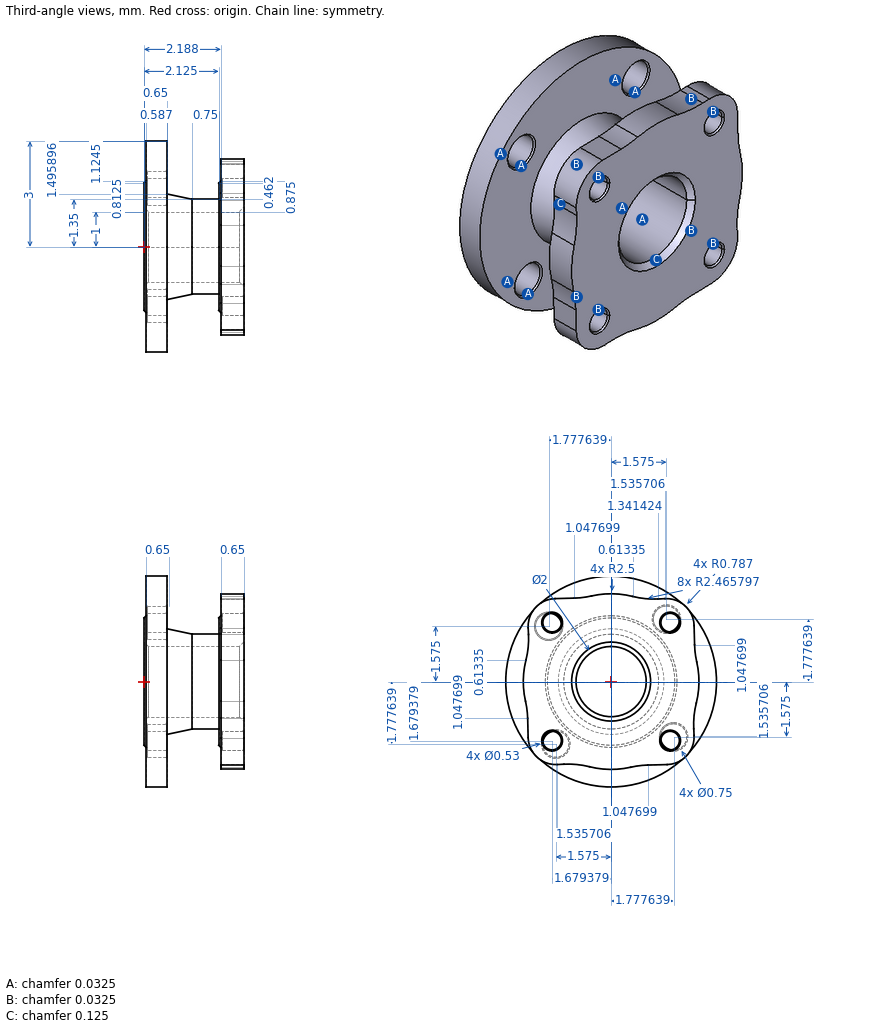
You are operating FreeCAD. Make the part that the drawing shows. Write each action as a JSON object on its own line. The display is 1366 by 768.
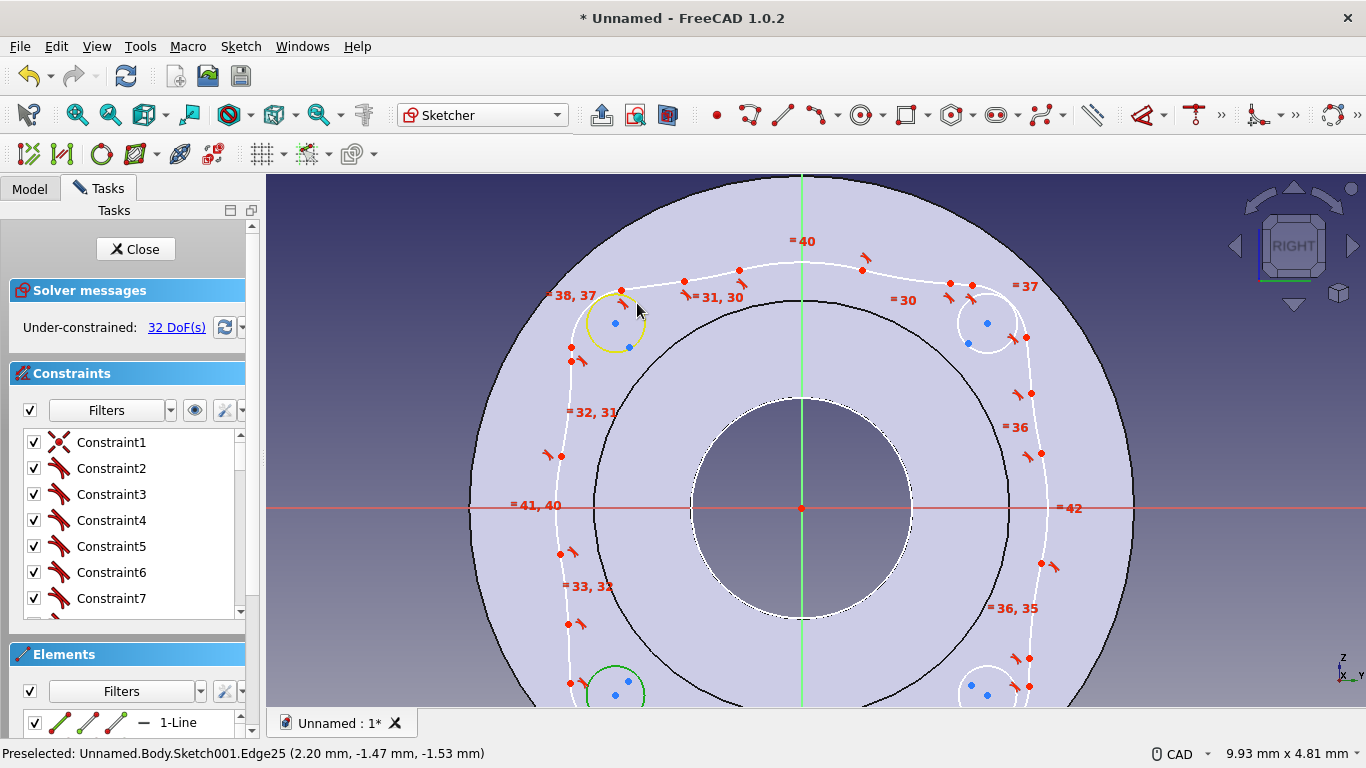
{"action": "left_click", "coordinate": [636, 303]}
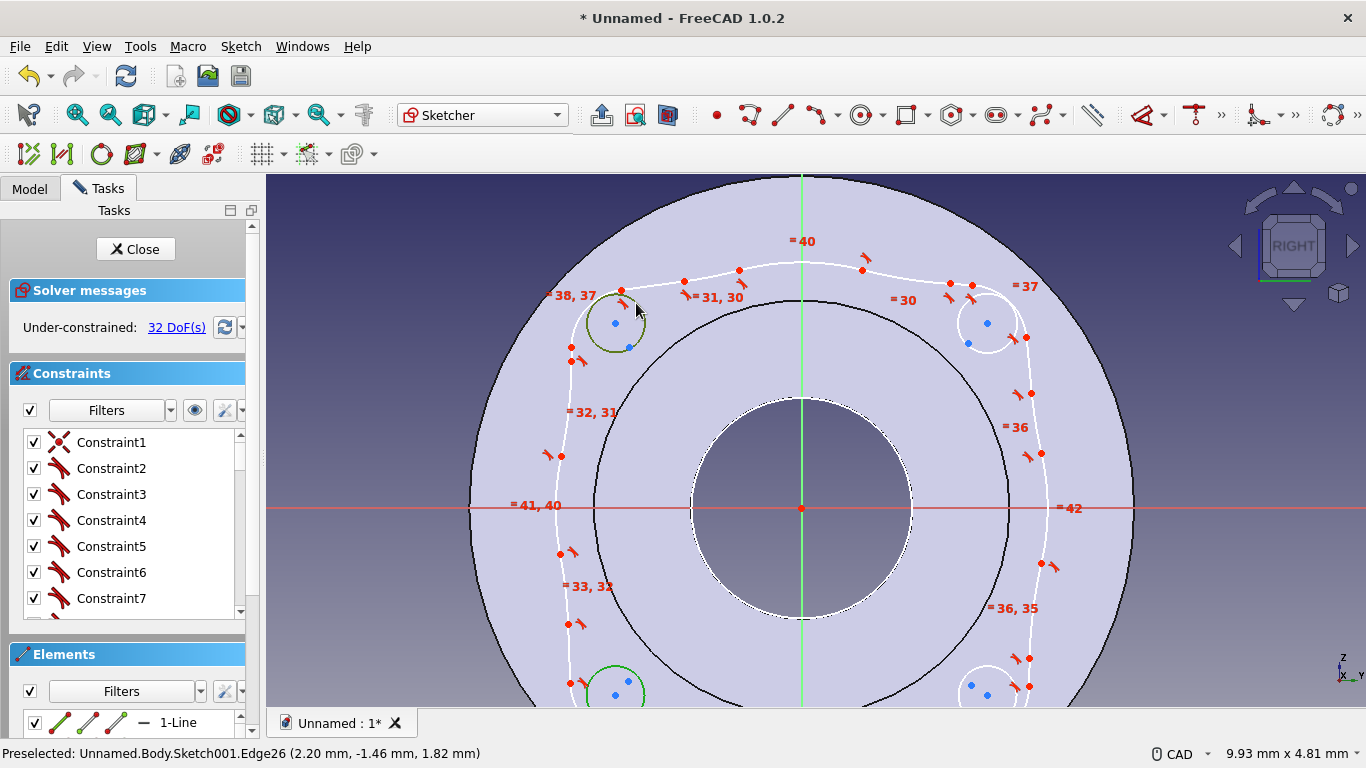
{"action": "left_click", "coordinate": [1008, 675]}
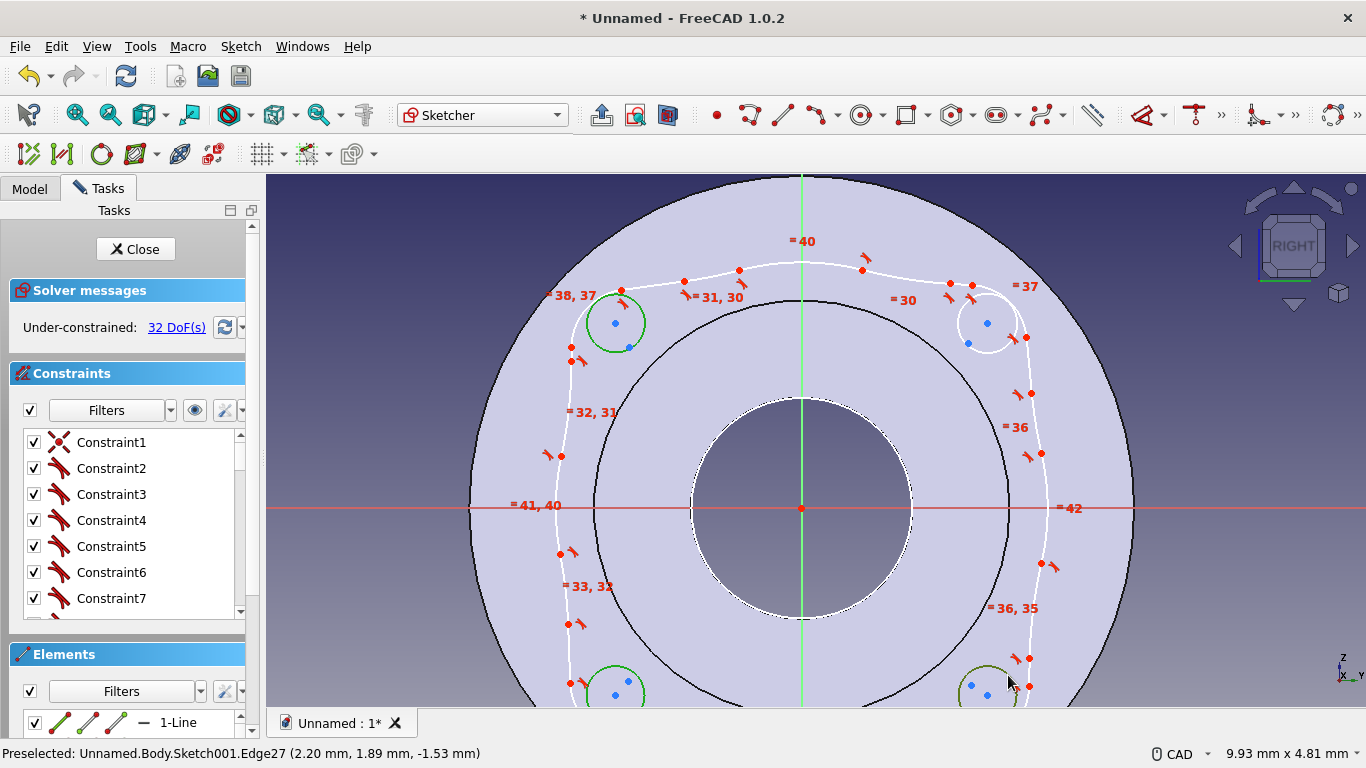
{"action": "left_click", "coordinate": [1009, 344]}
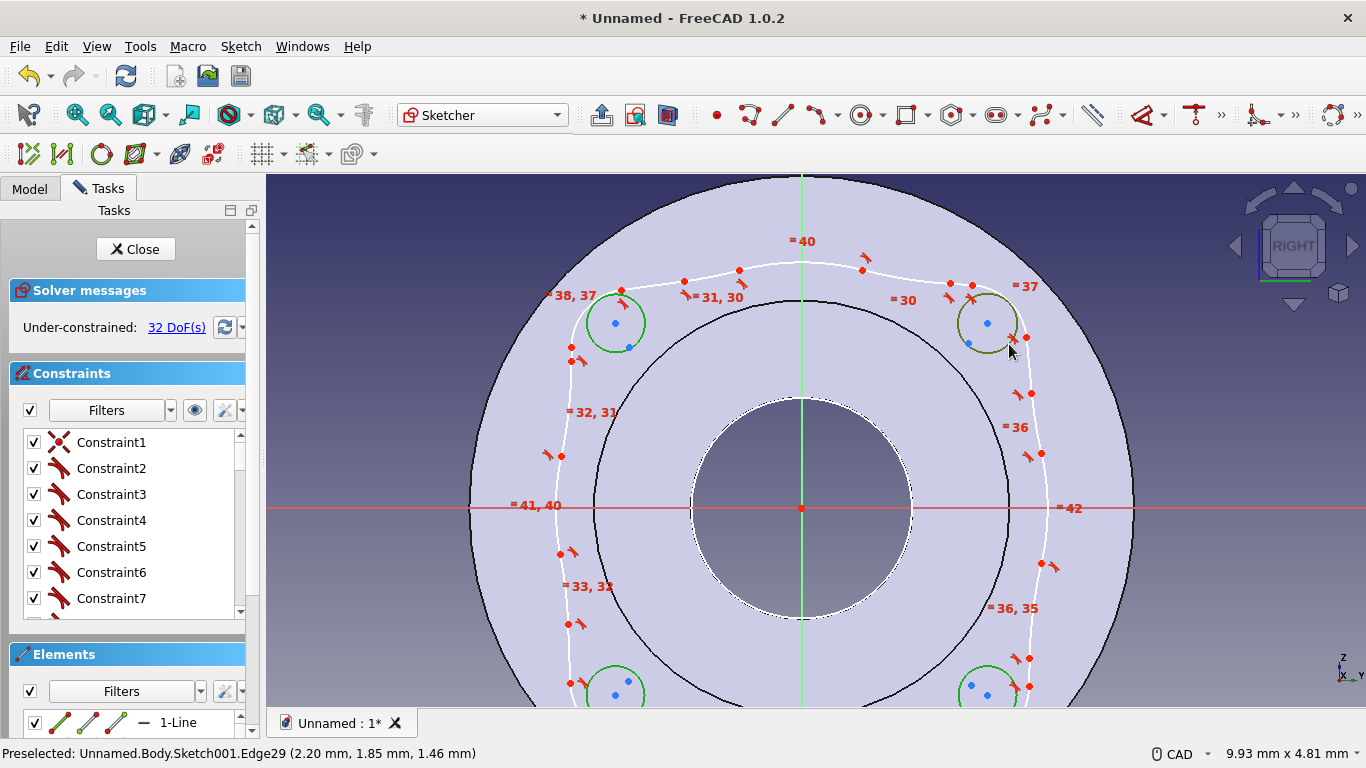
{"action": "key", "text": "e"}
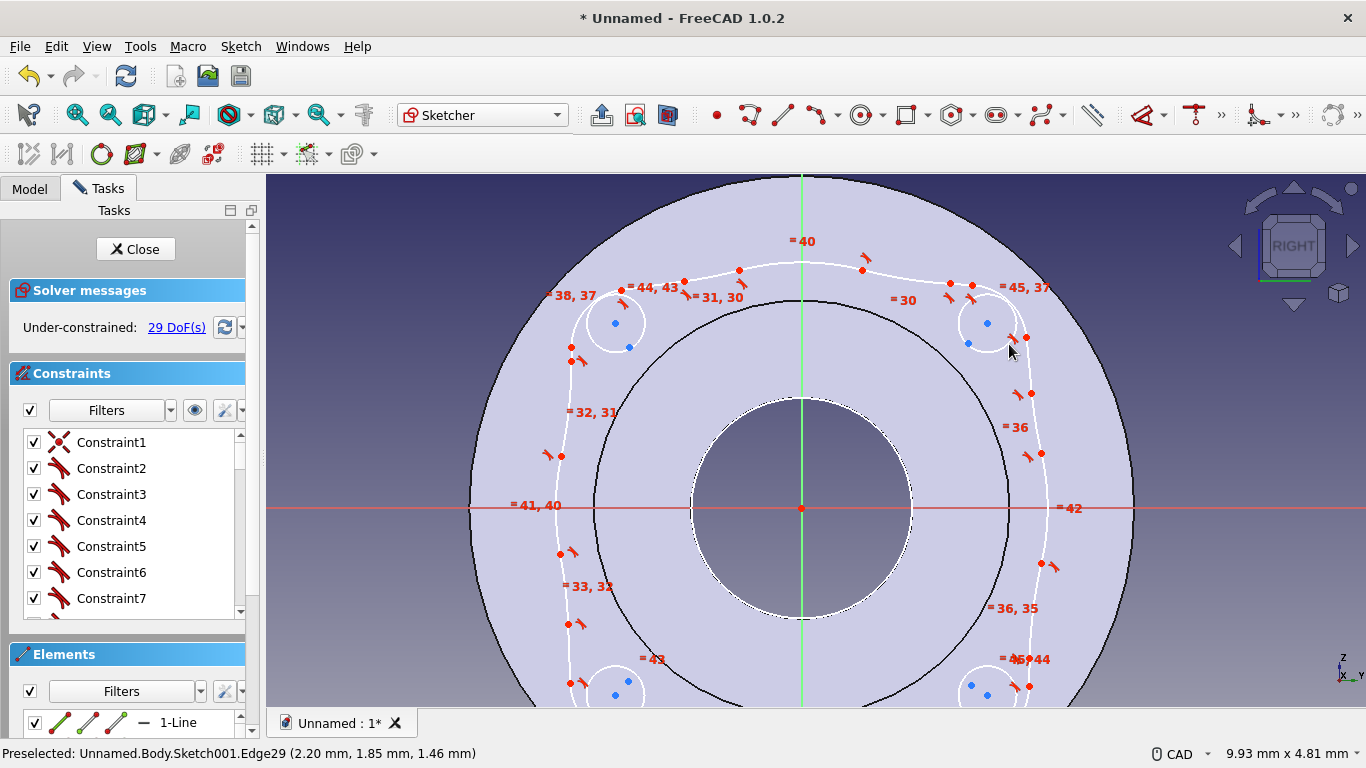
{"action": "left_click", "coordinate": [969, 343]}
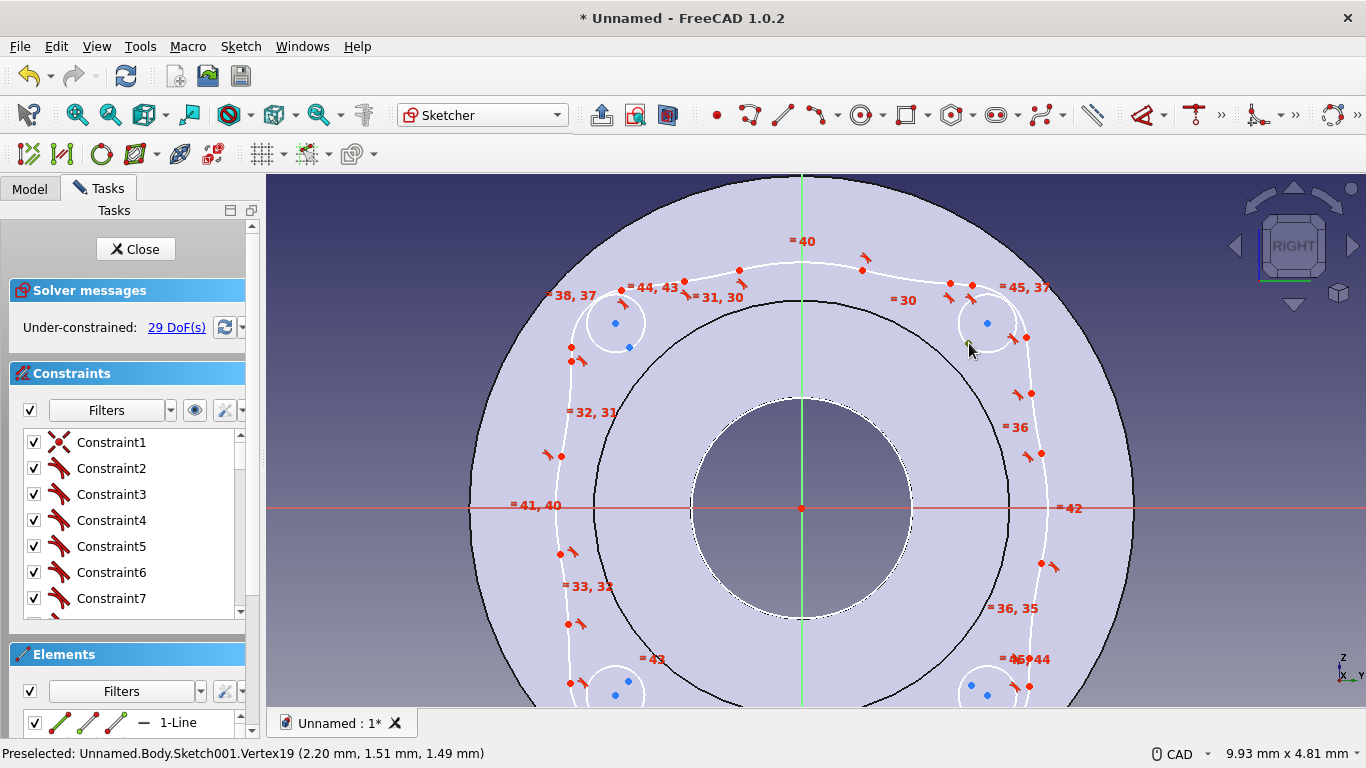
{"action": "left_click", "coordinate": [630, 347]}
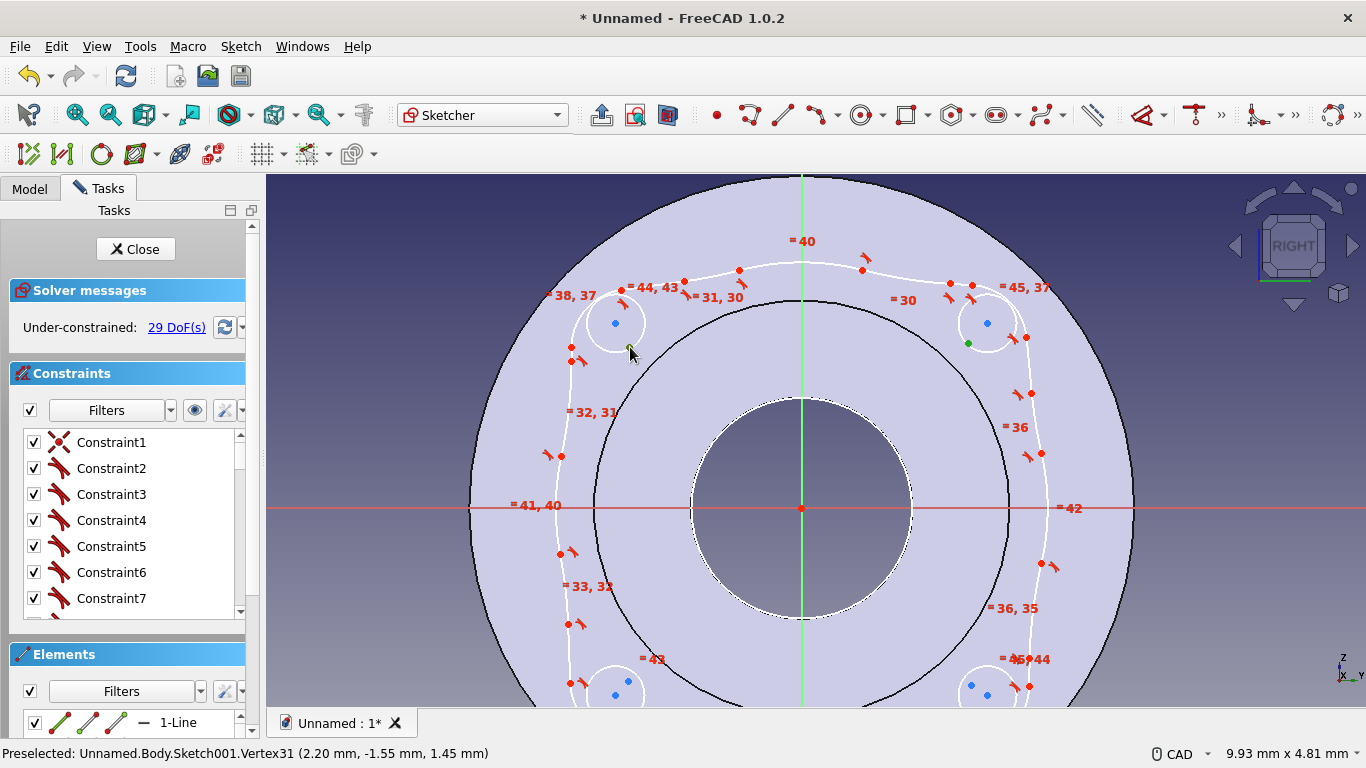
{"action": "left_click", "coordinate": [802, 577]}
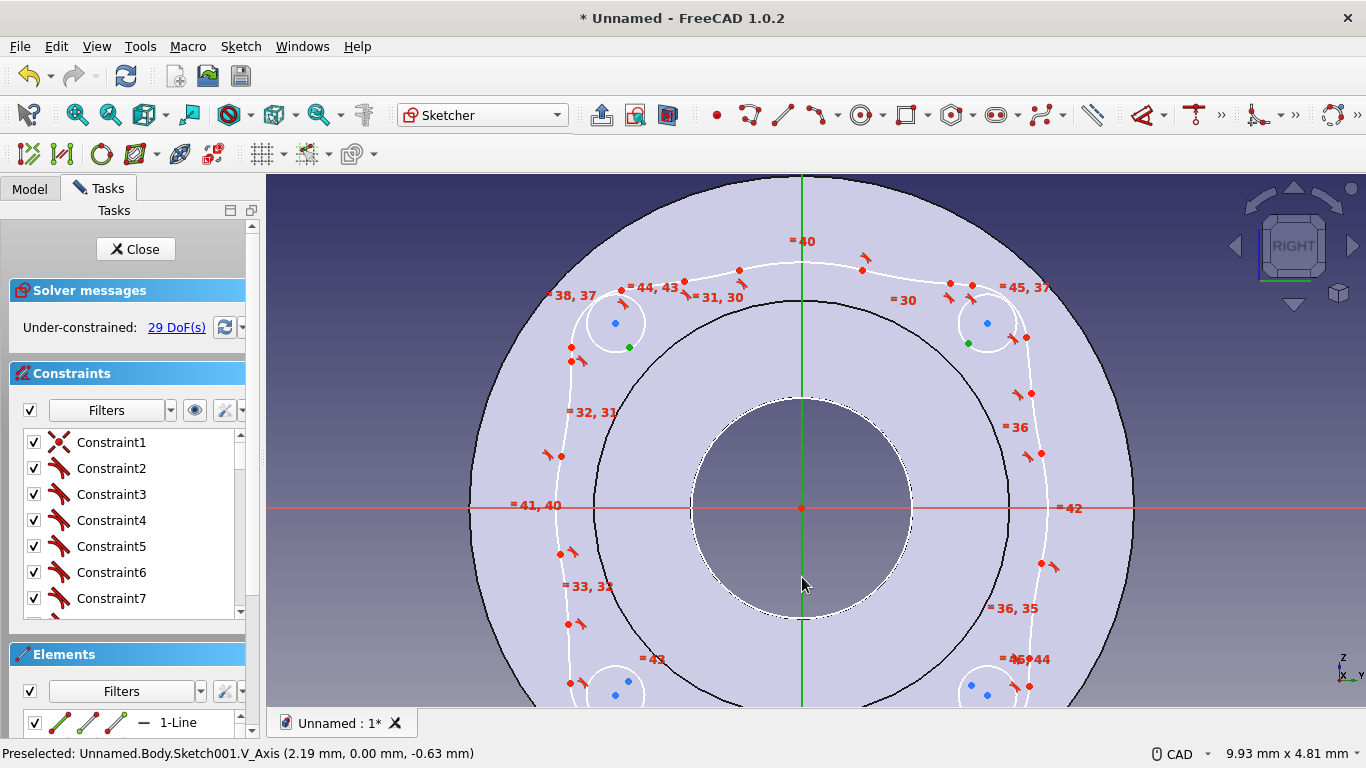
{"action": "key", "text": "s"}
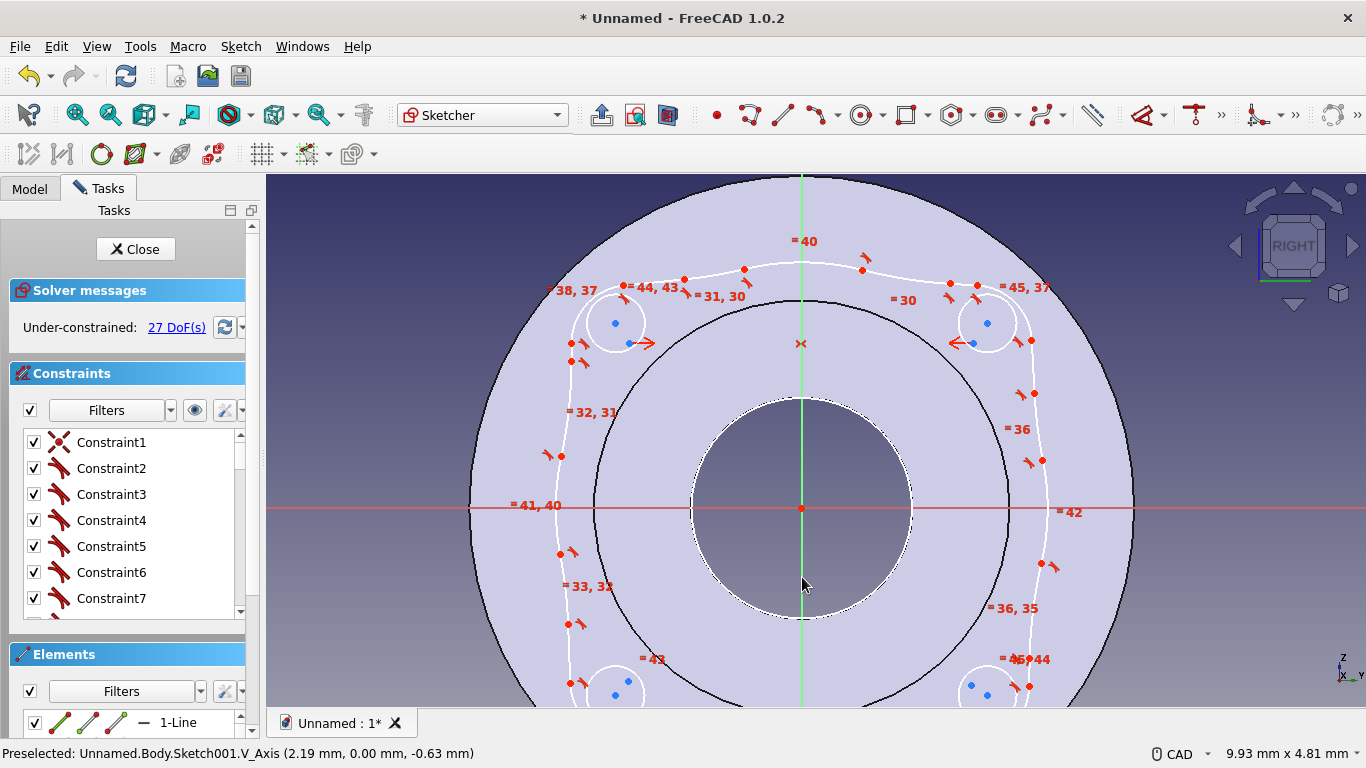
{"action": "left_click", "coordinate": [630, 343]}